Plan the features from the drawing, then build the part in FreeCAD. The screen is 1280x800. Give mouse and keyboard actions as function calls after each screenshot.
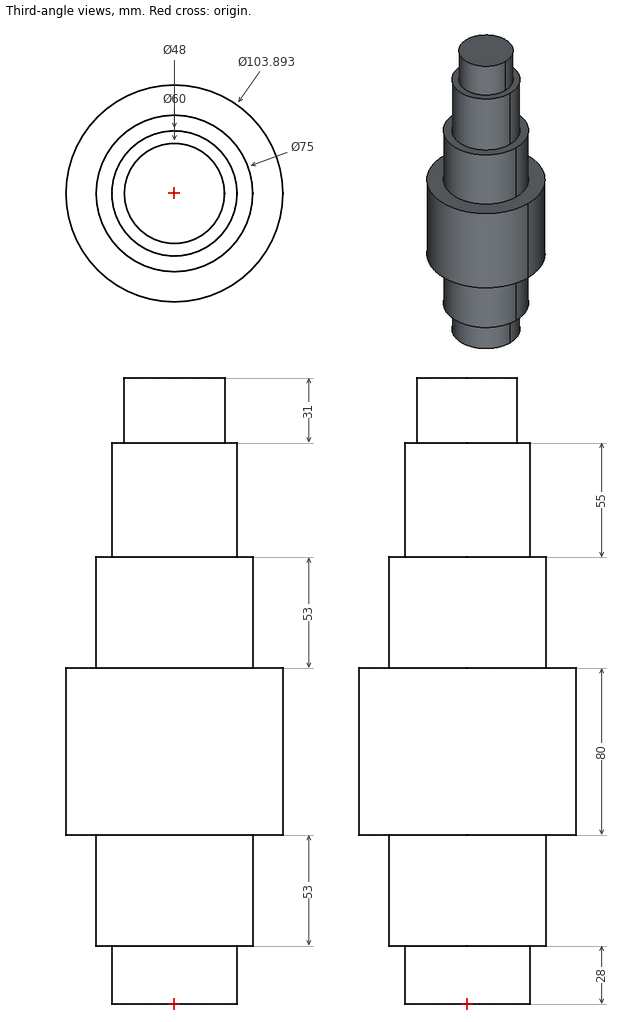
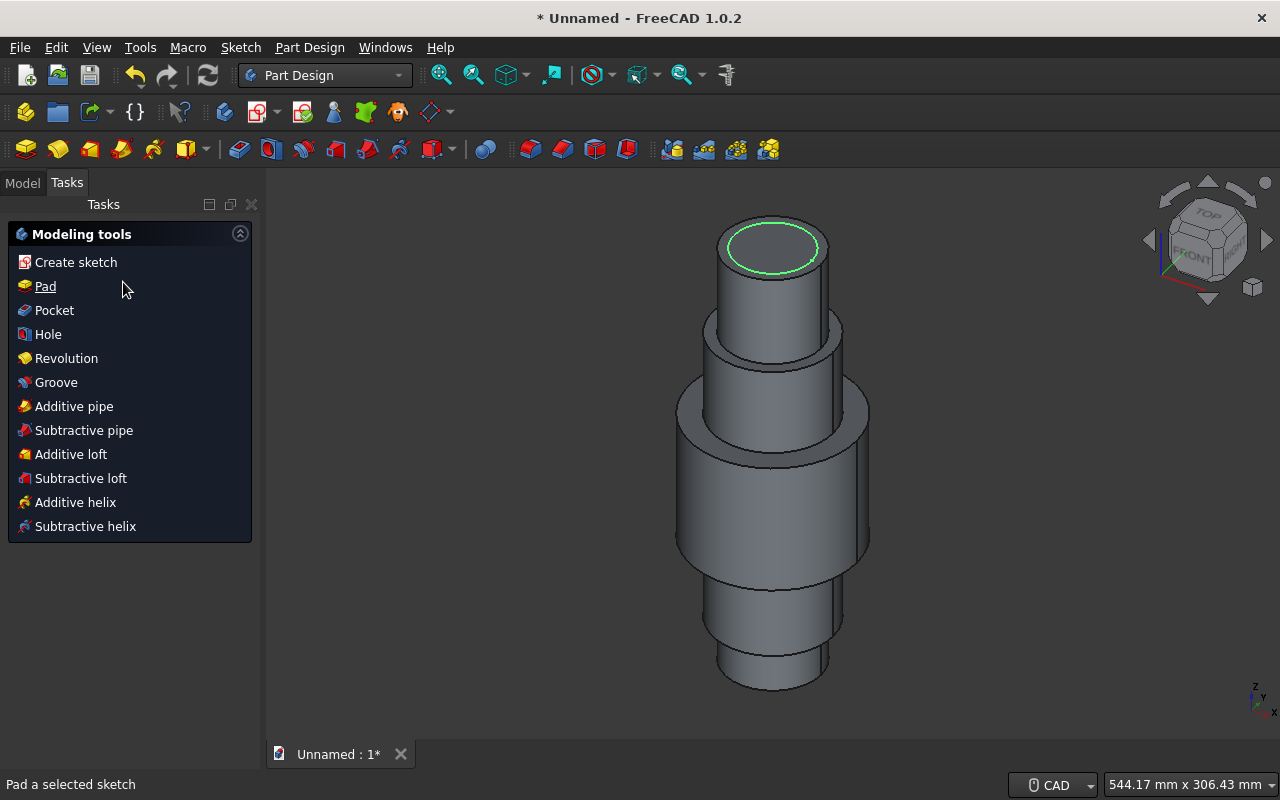
click(26, 150)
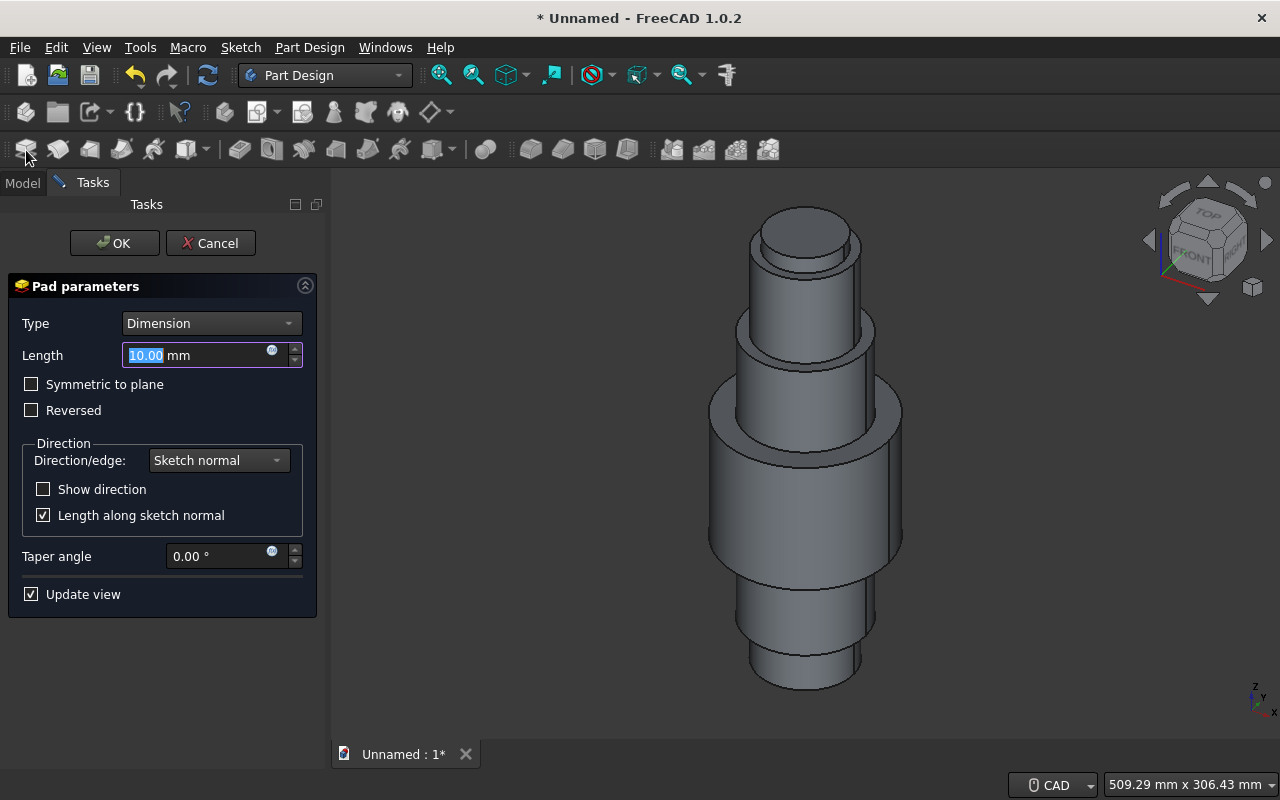
text(31)
key(Tab)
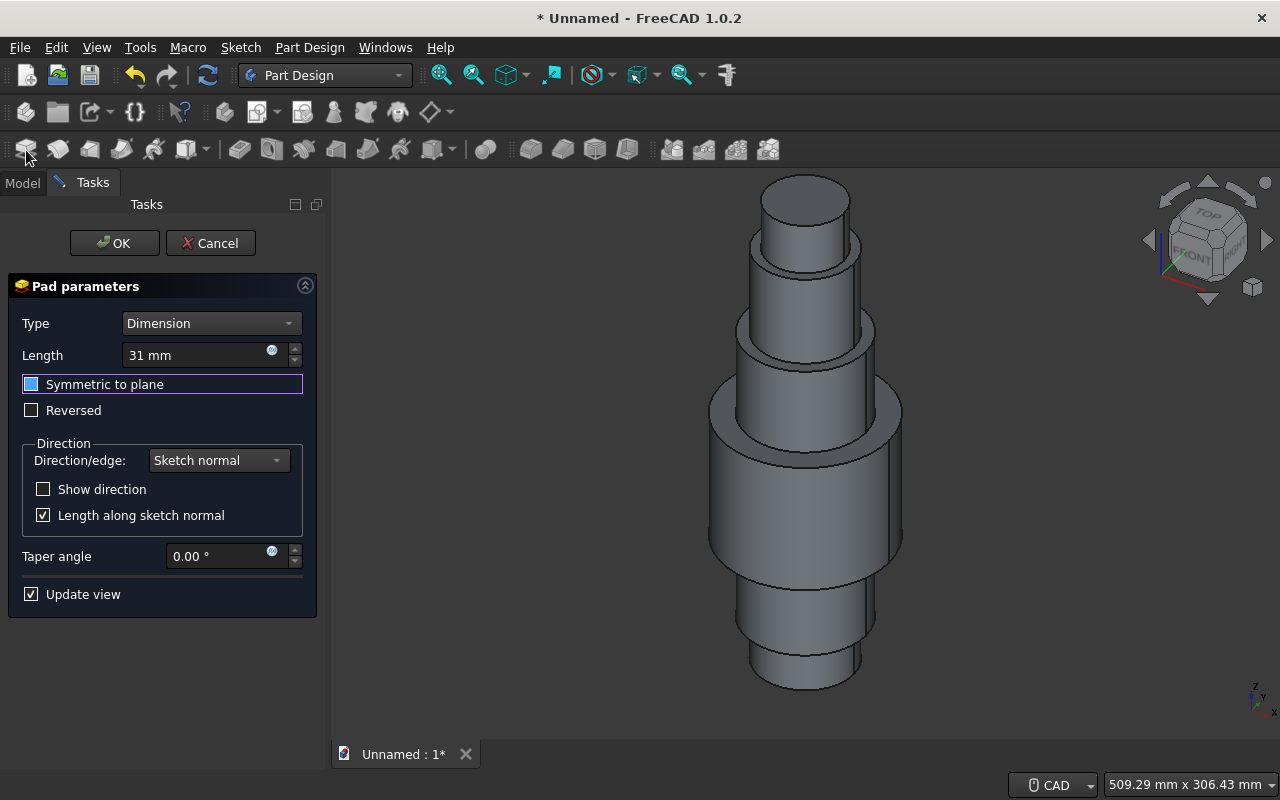
click(115, 243)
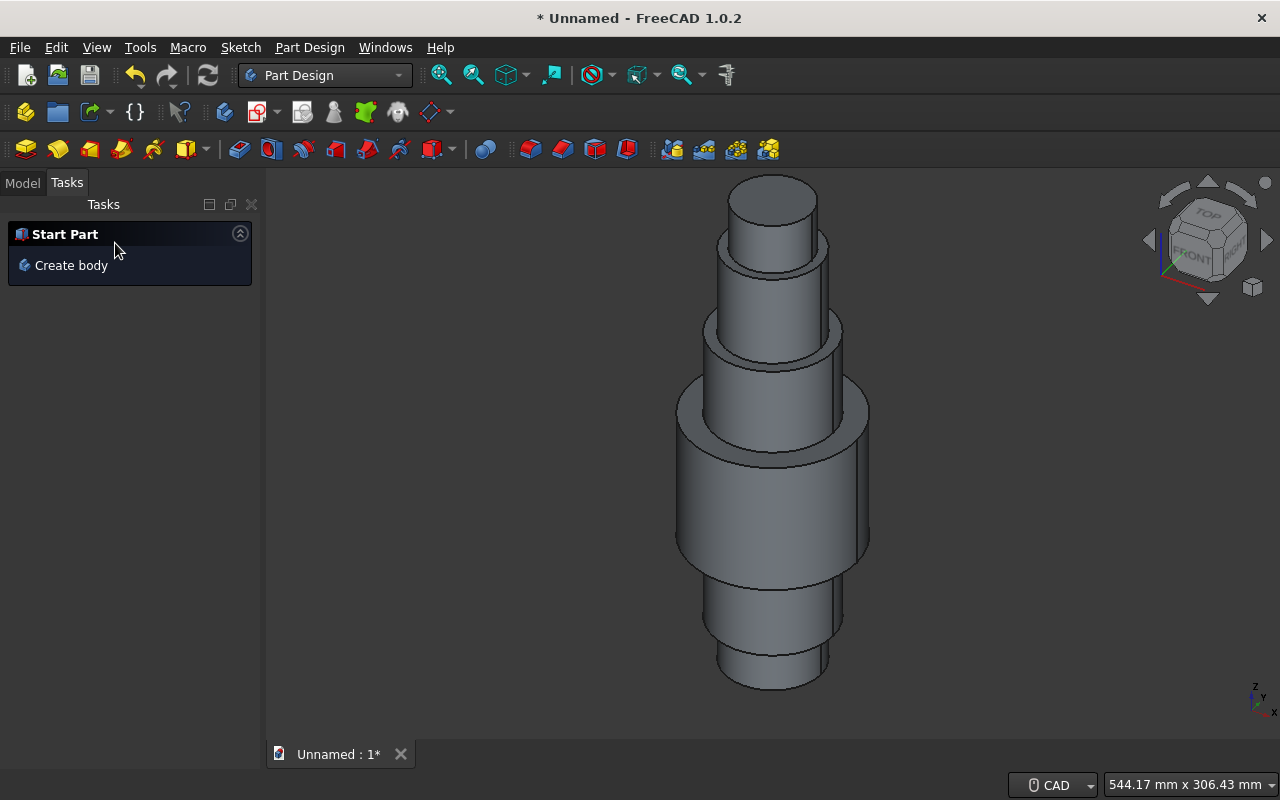
key(0)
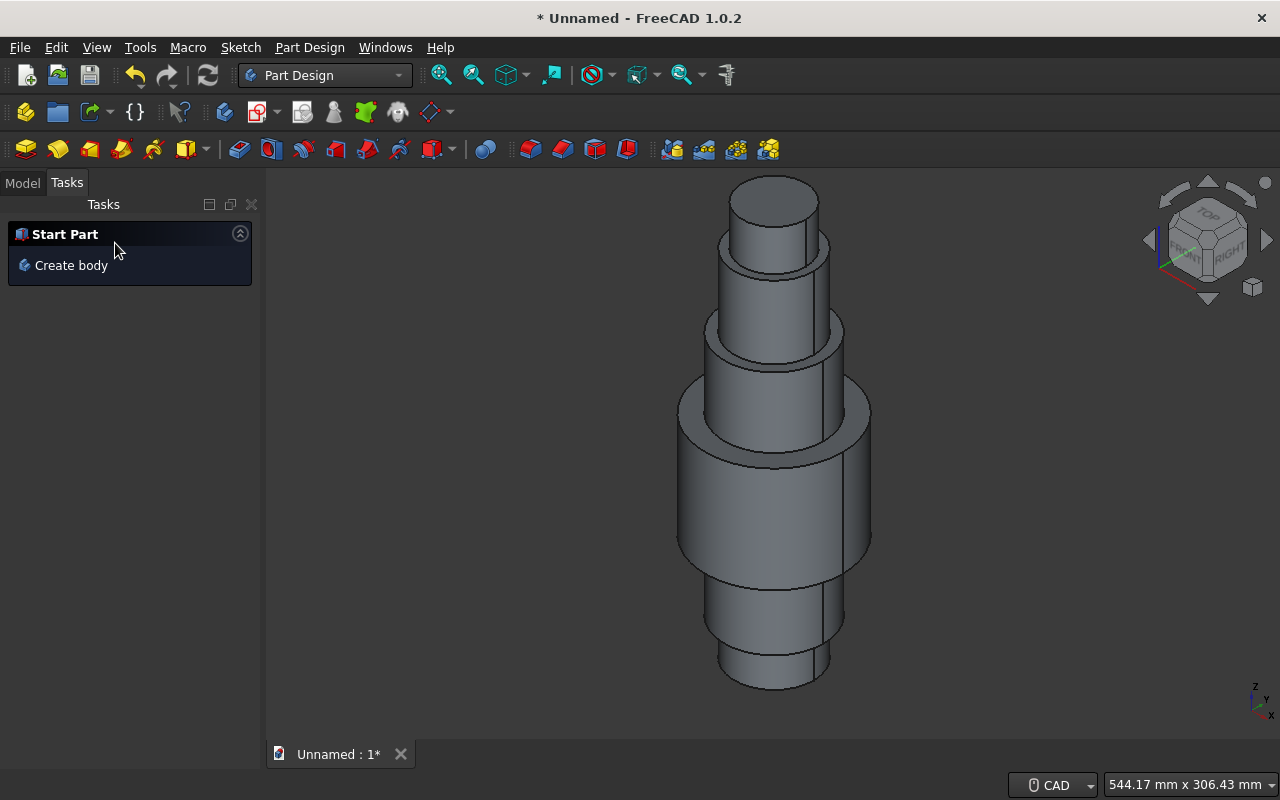
click(442, 76)